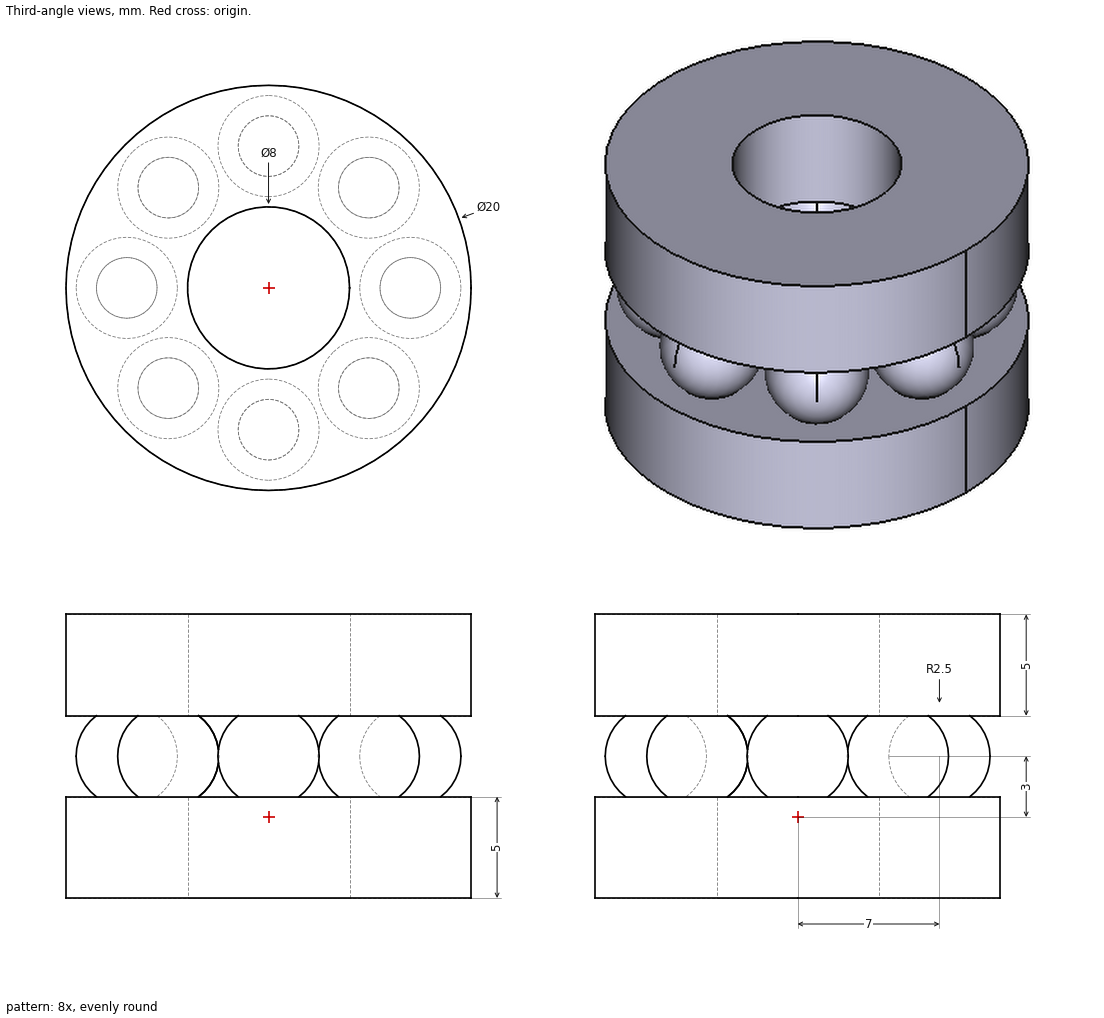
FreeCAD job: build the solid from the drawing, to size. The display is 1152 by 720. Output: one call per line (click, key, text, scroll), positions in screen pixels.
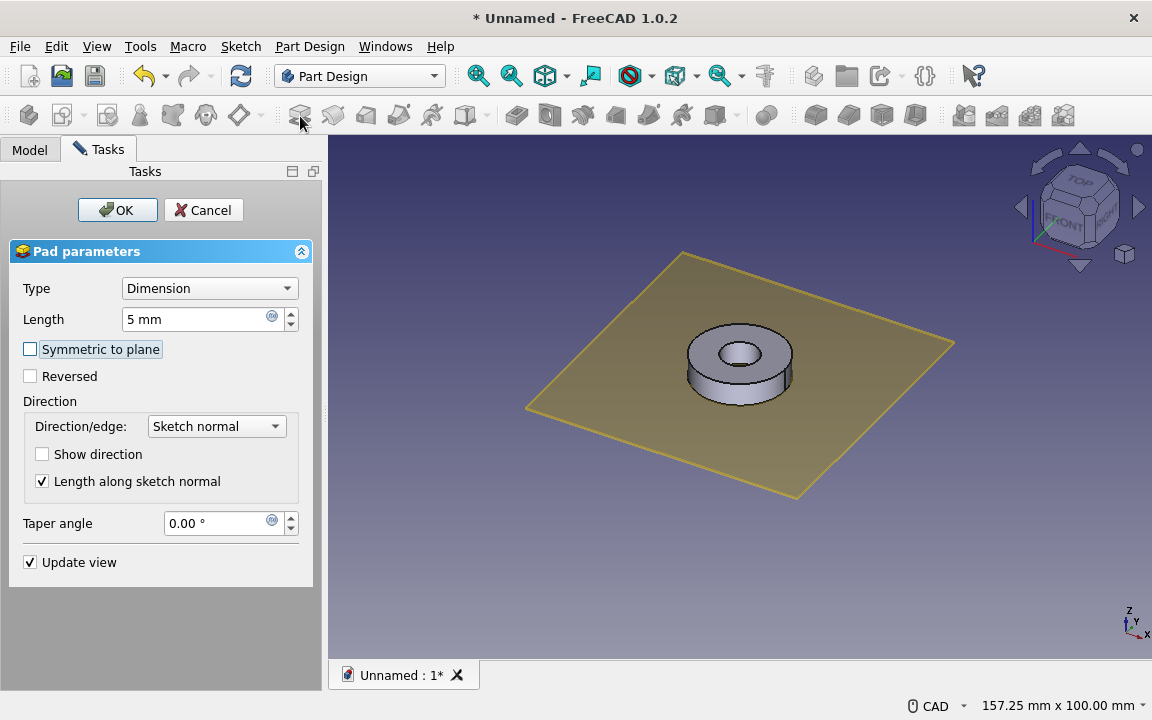
click(118, 210)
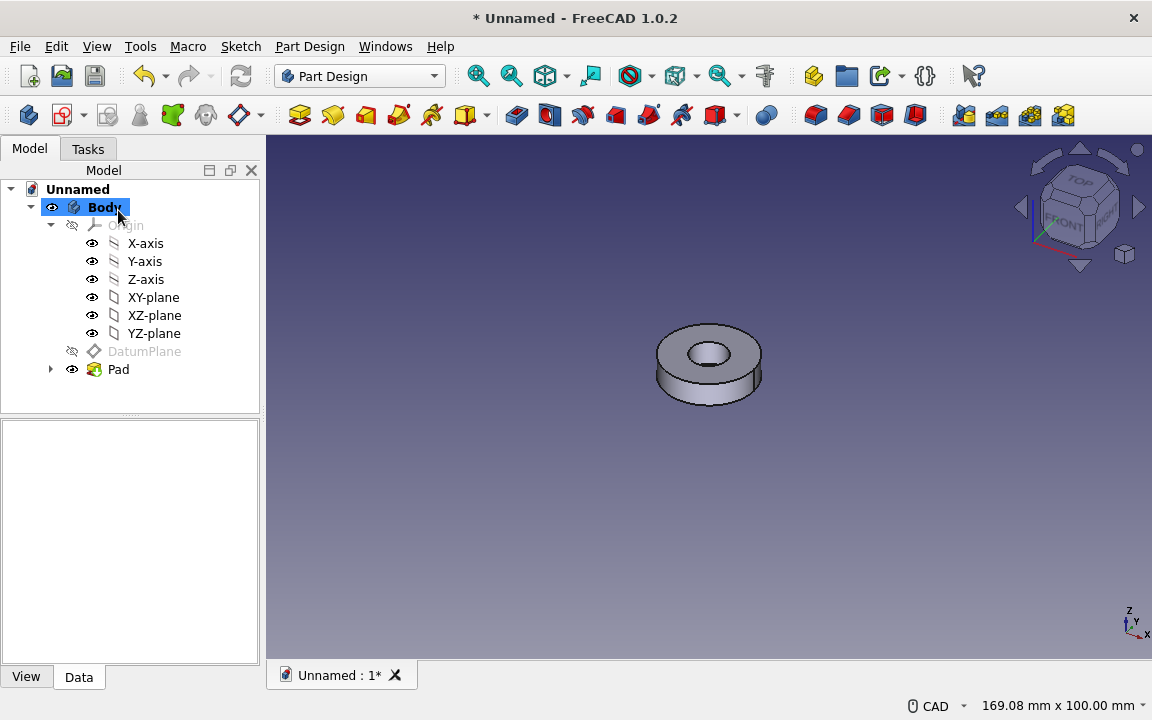
click(479, 76)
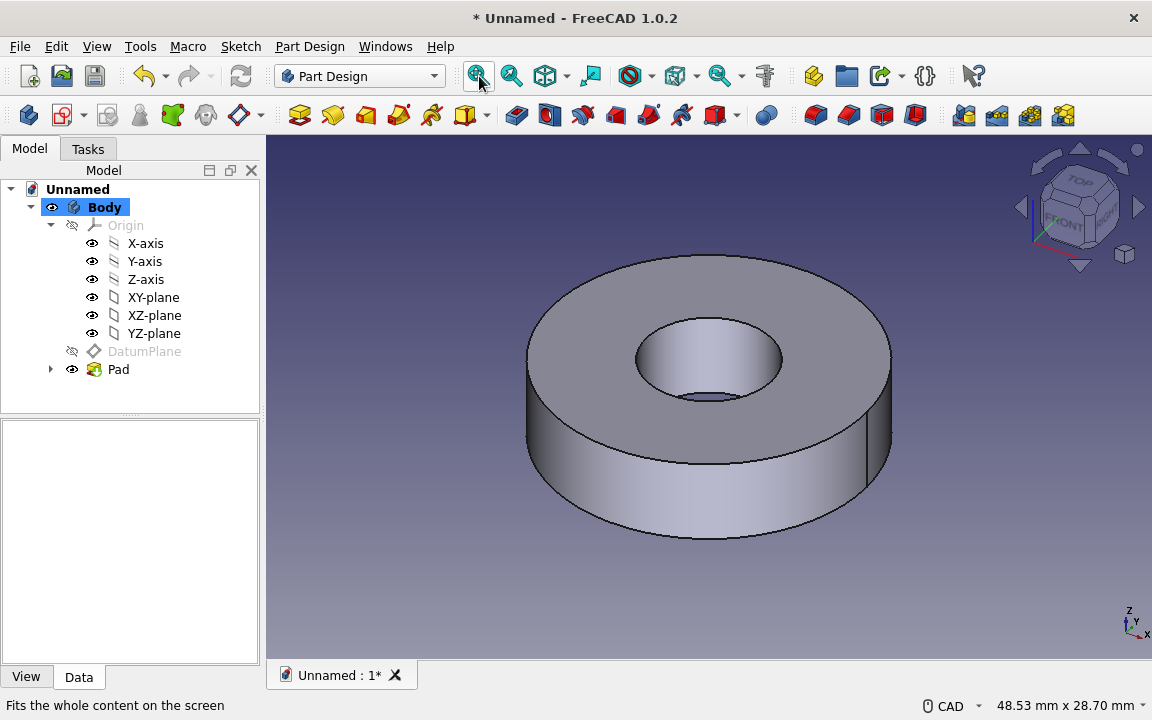
click(62, 116)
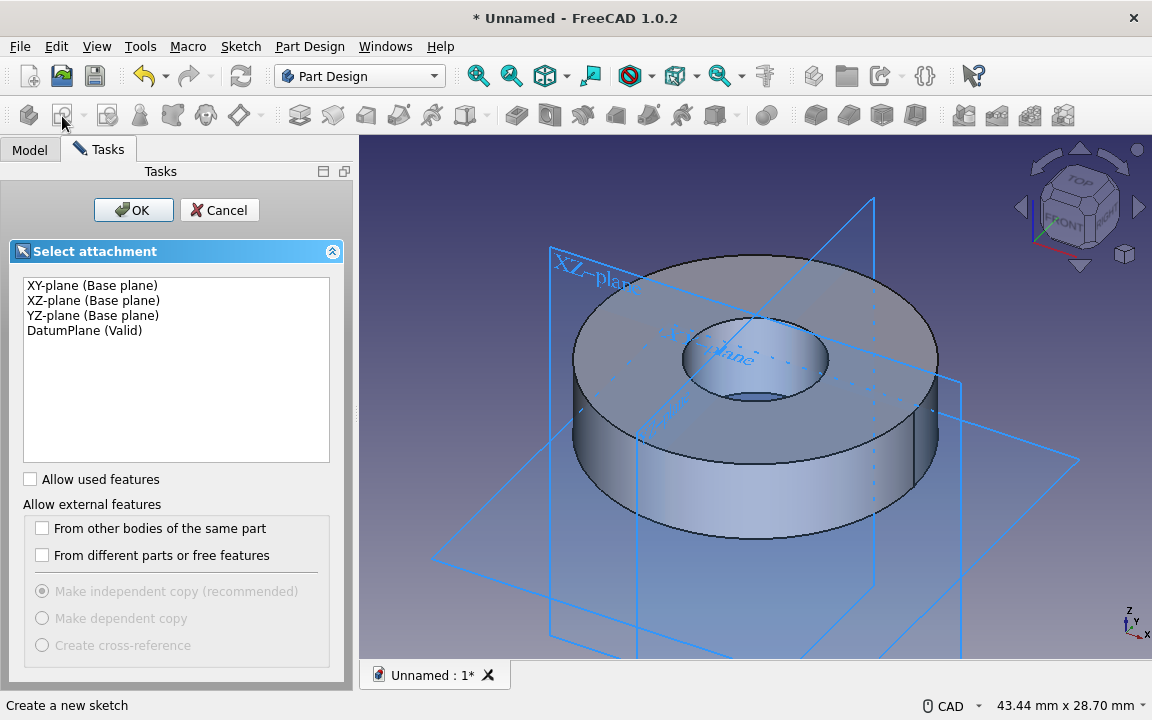
click(84, 316)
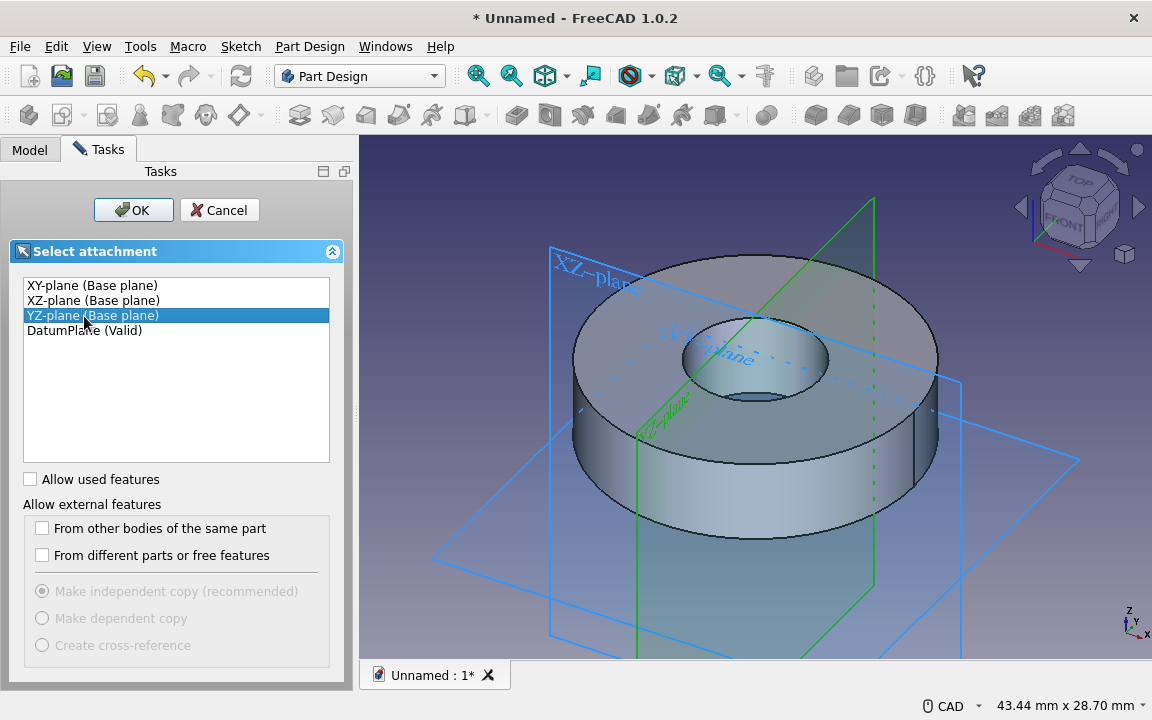
click(134, 210)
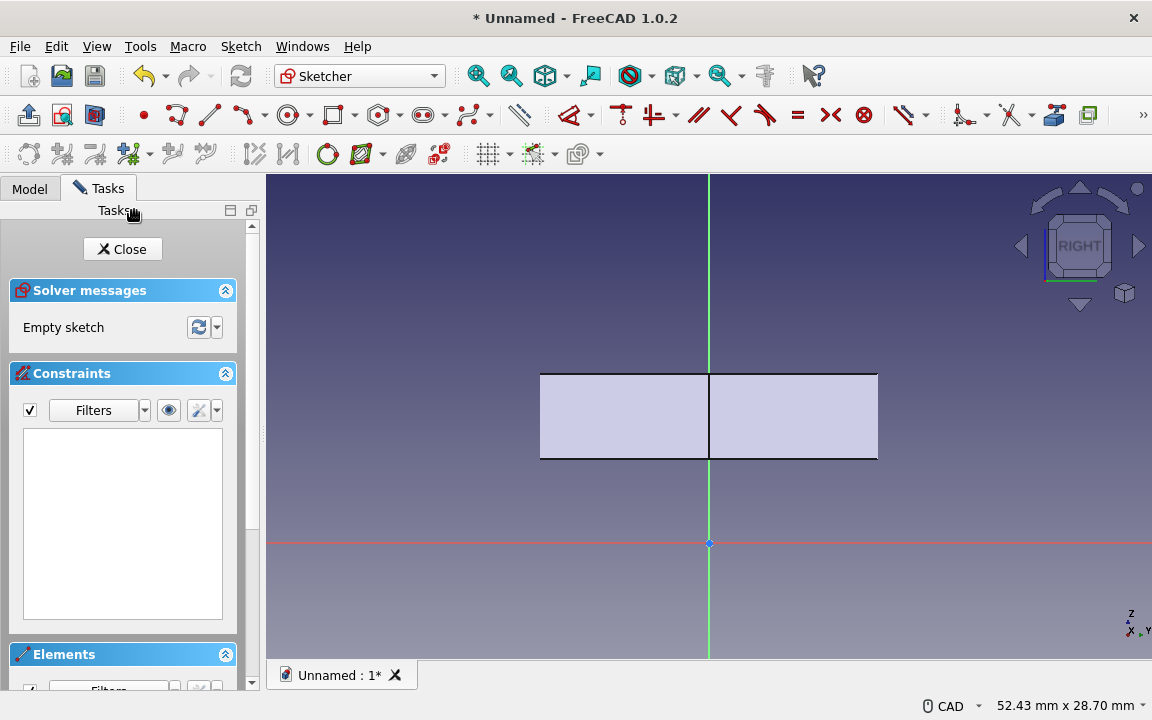
click(95, 116)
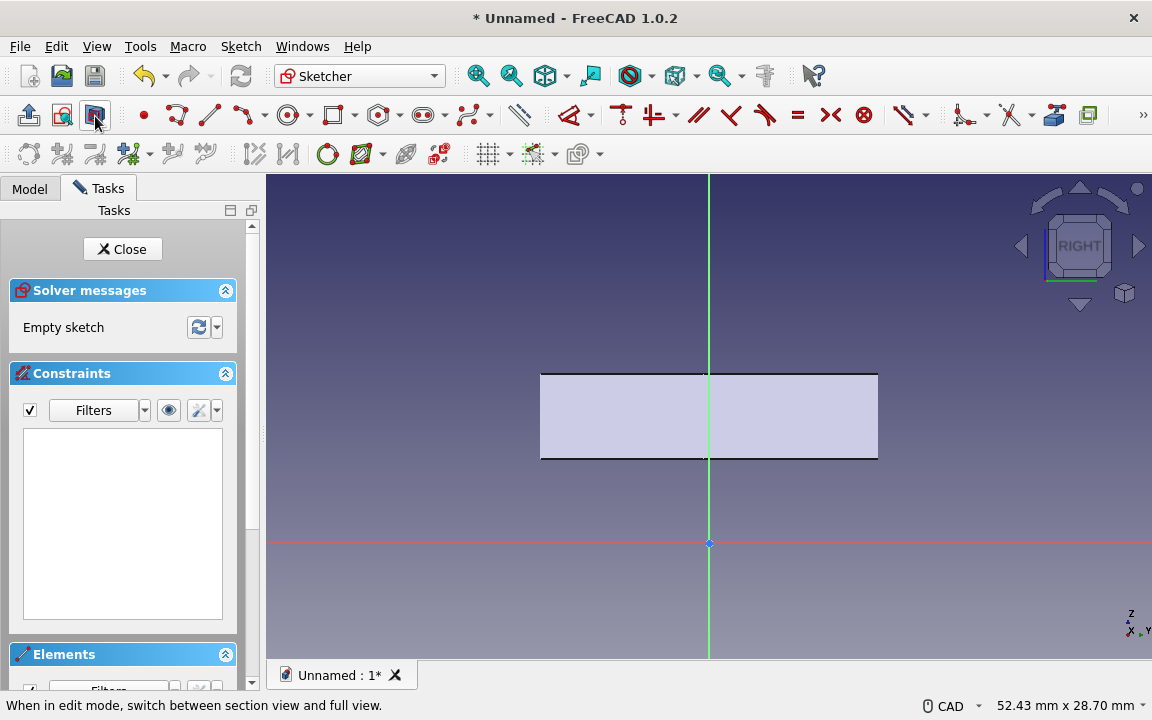
scroll(903, 543, up, 5)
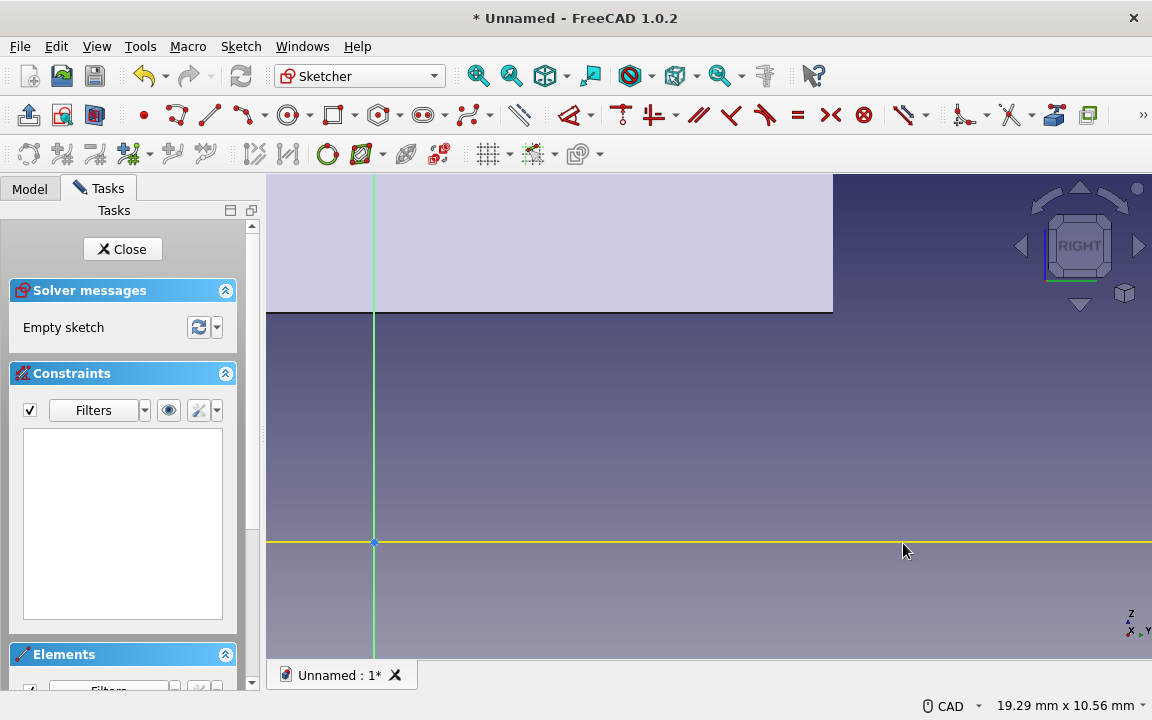
click(210, 116)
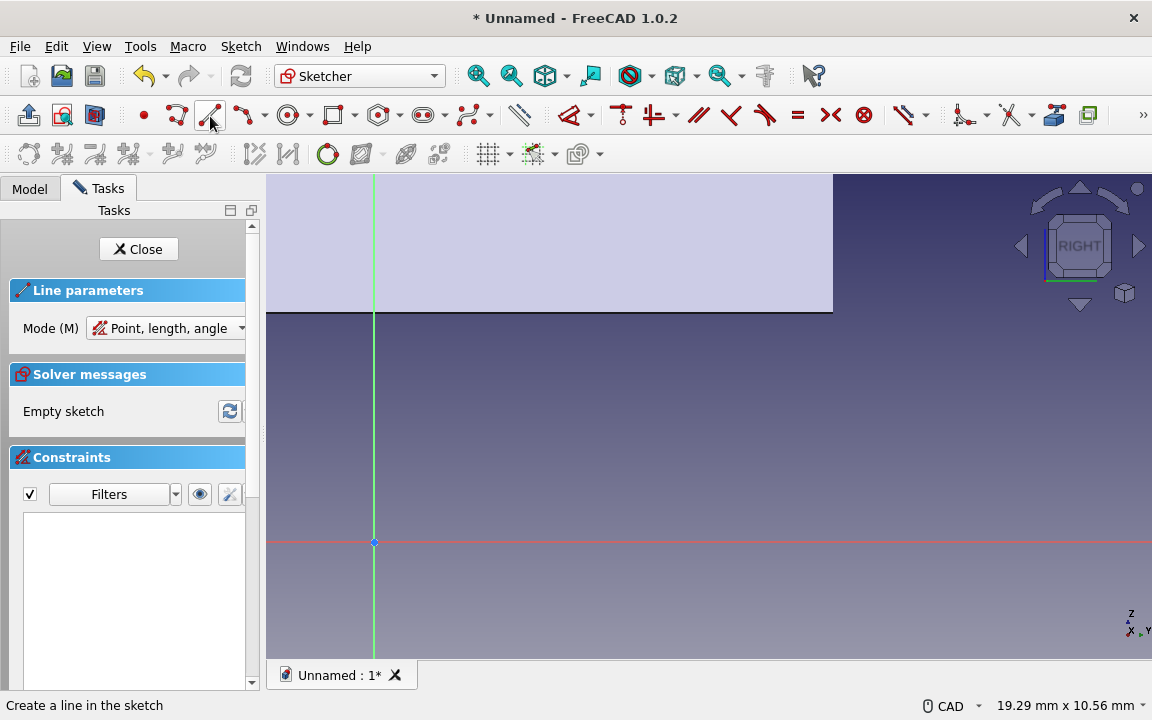
click(581, 405)
click(811, 405)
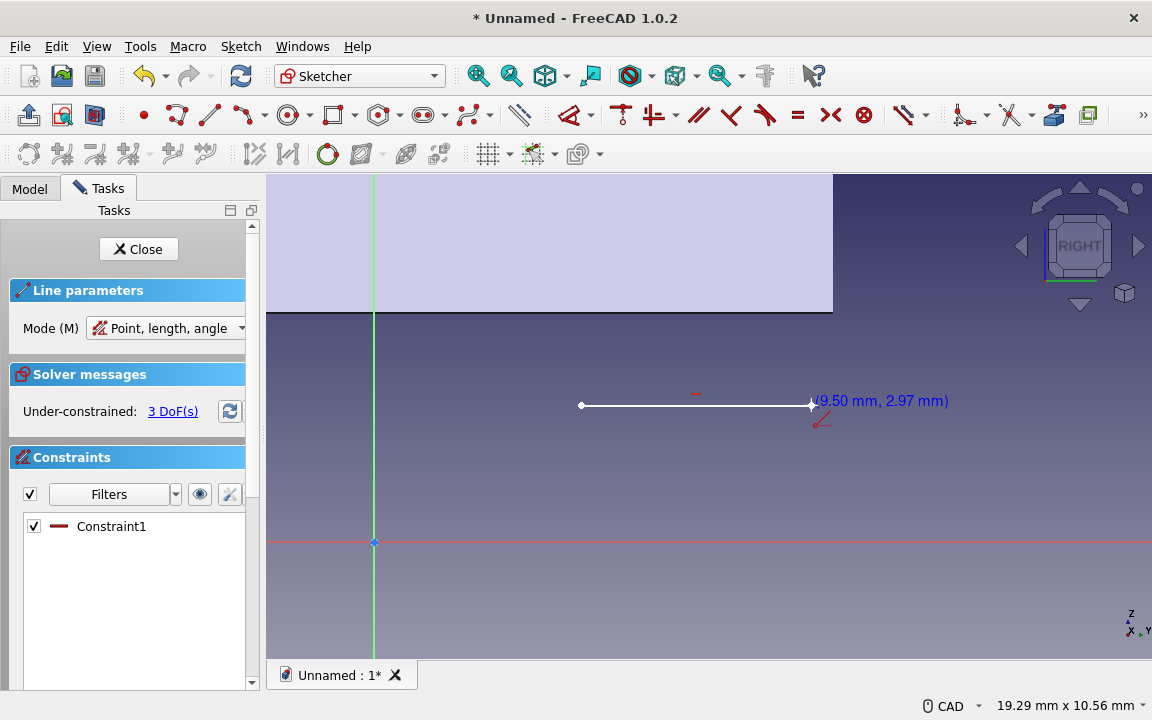
click(242, 116)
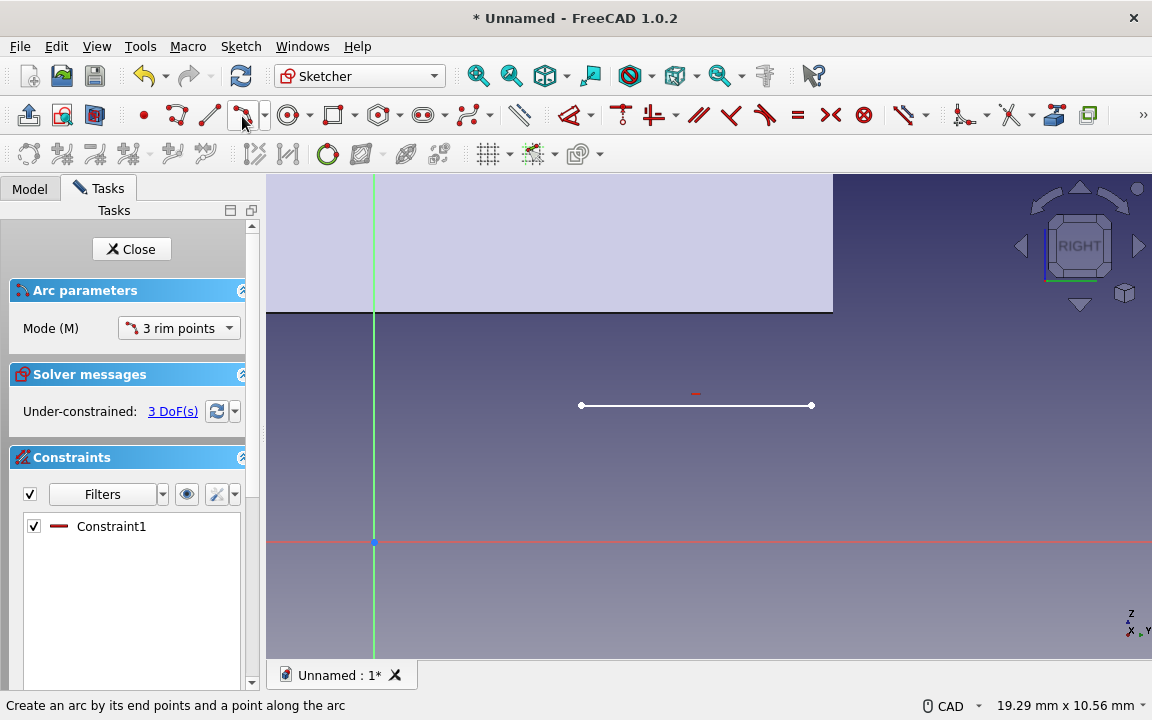
click(811, 406)
click(581, 406)
click(696, 290)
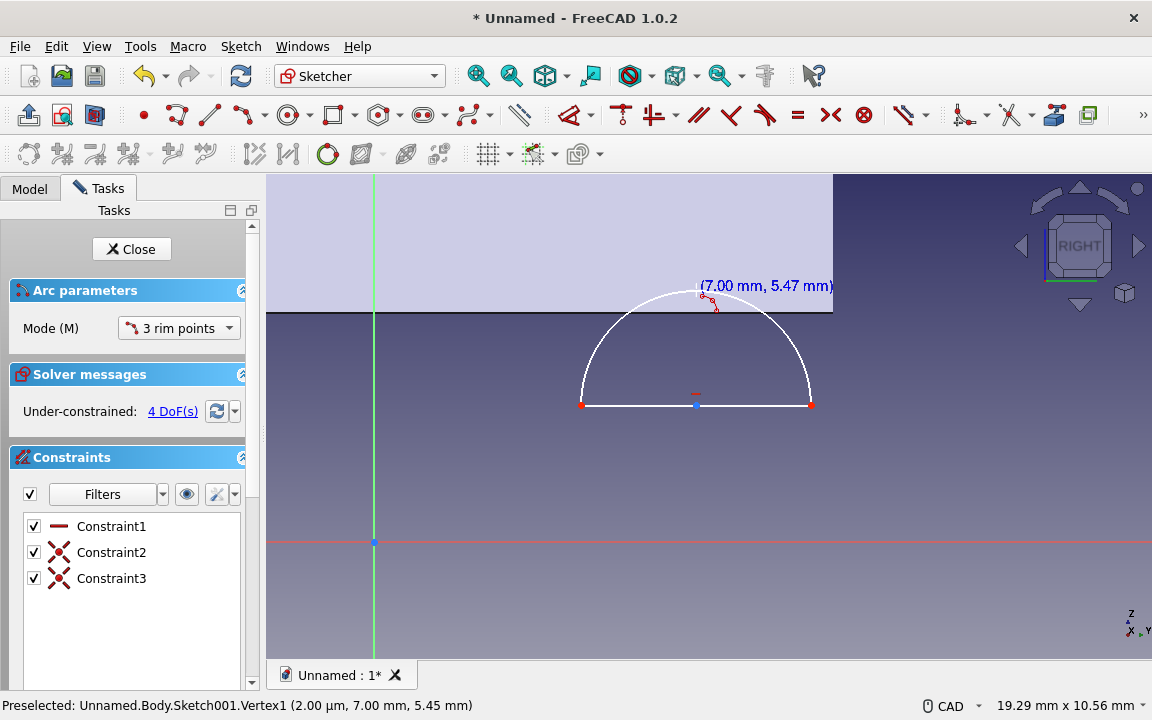
click(210, 116)